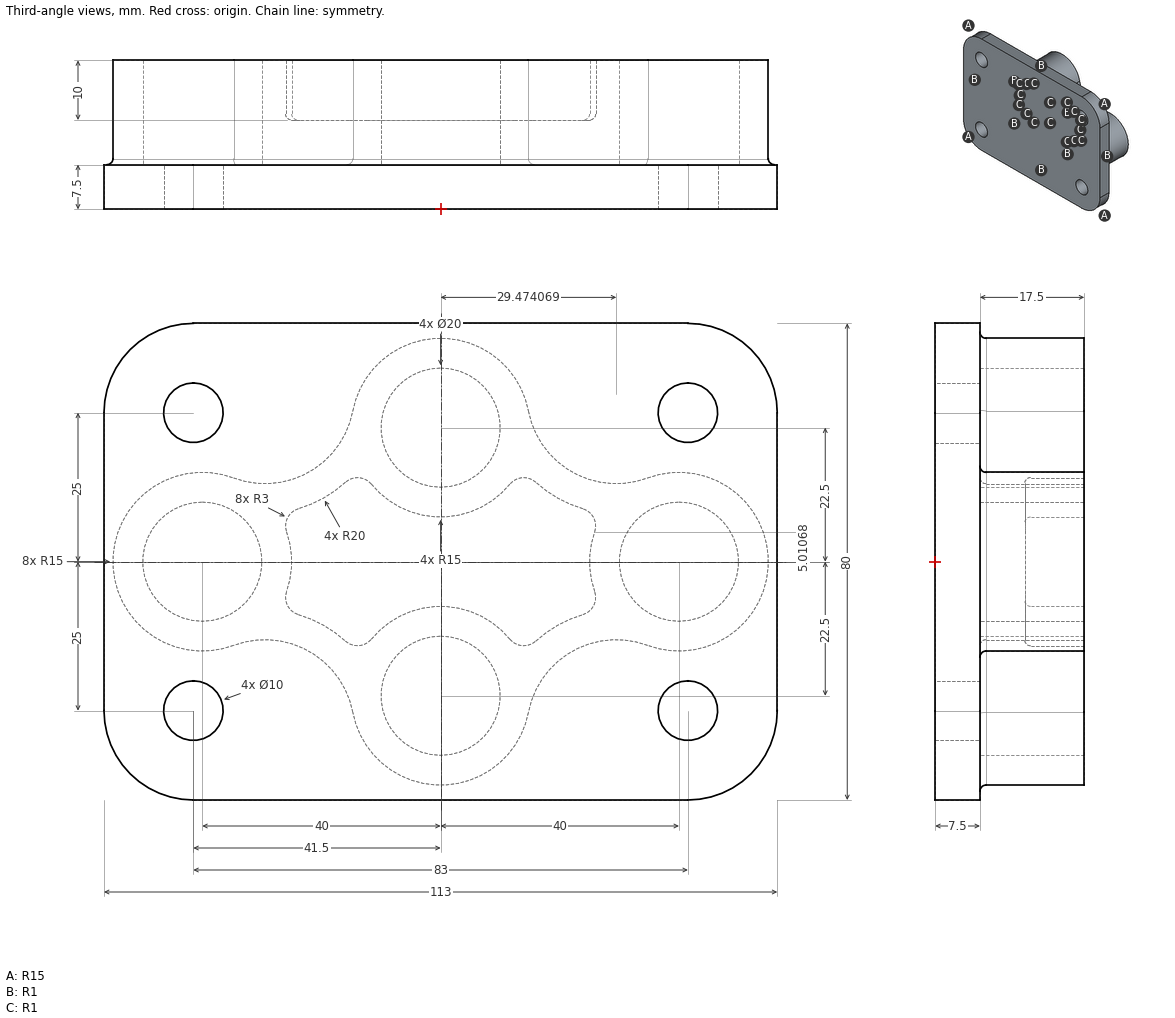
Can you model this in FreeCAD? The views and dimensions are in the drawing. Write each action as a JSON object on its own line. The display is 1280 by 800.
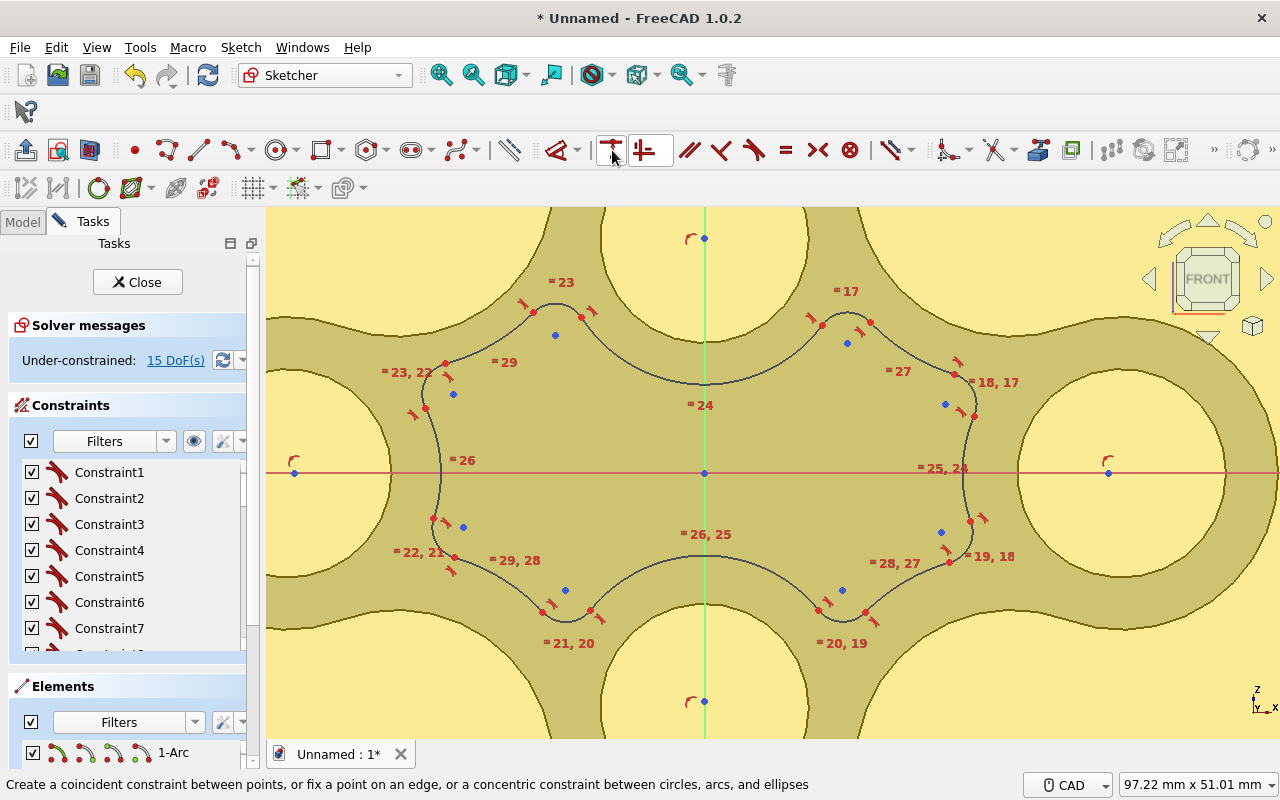
{"action": "scroll", "coordinate": [618, 711], "scroll_direction": "down", "scroll_amount": 1}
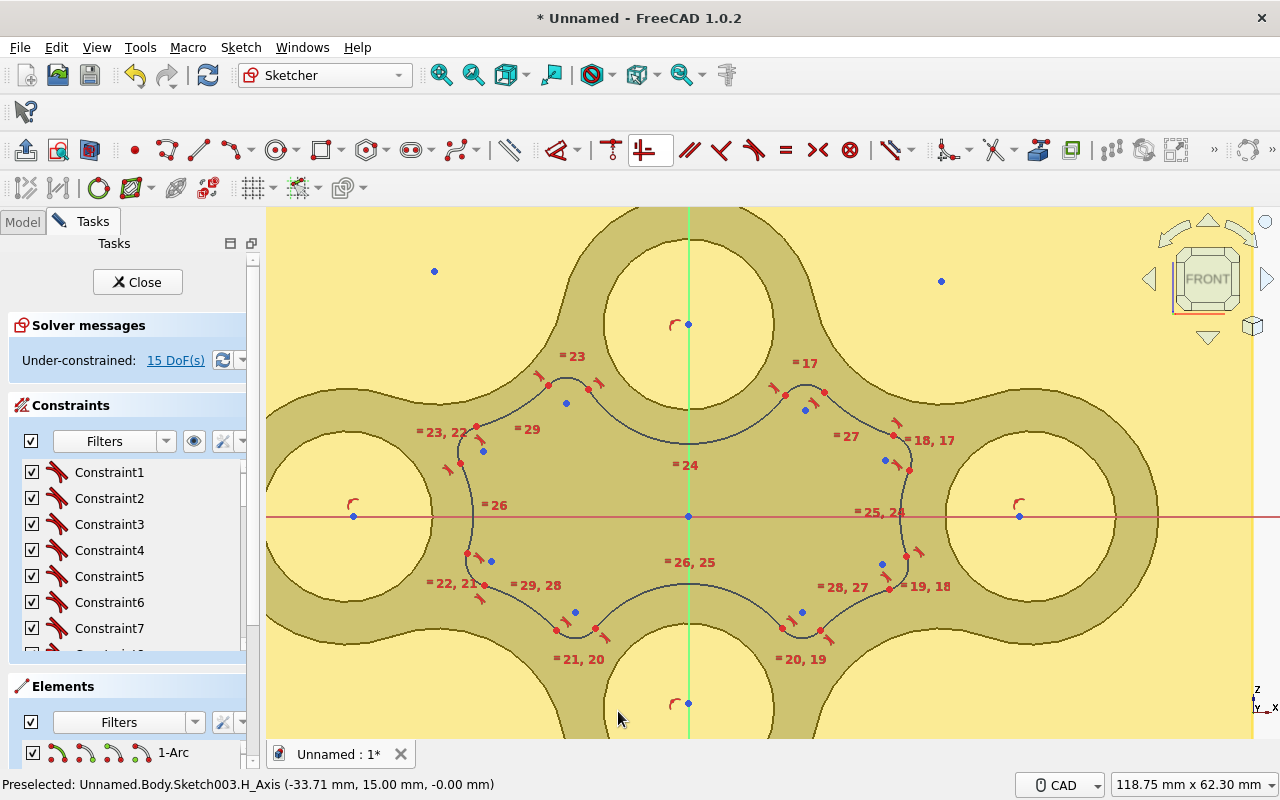
{"action": "left_click", "coordinate": [941, 282]}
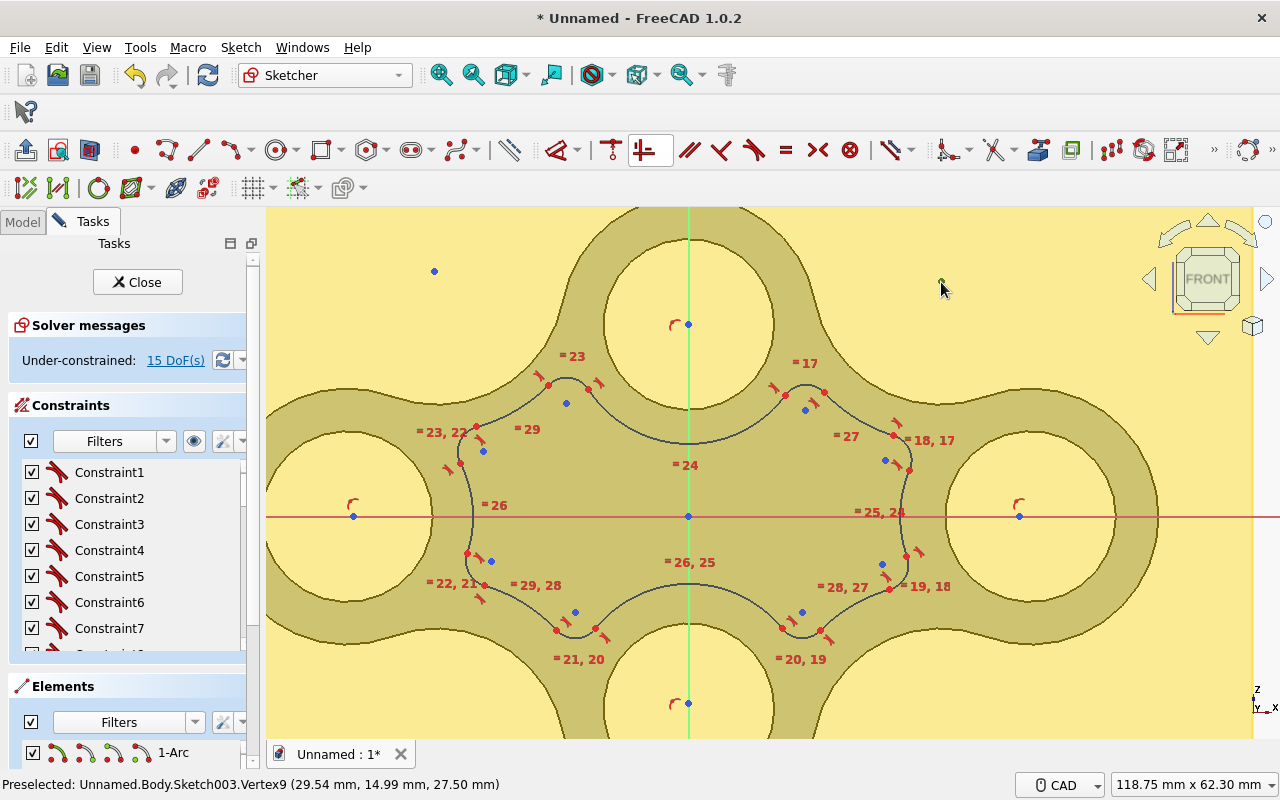
{"action": "scroll", "coordinate": [719, 235], "scroll_direction": "down", "scroll_amount": 1}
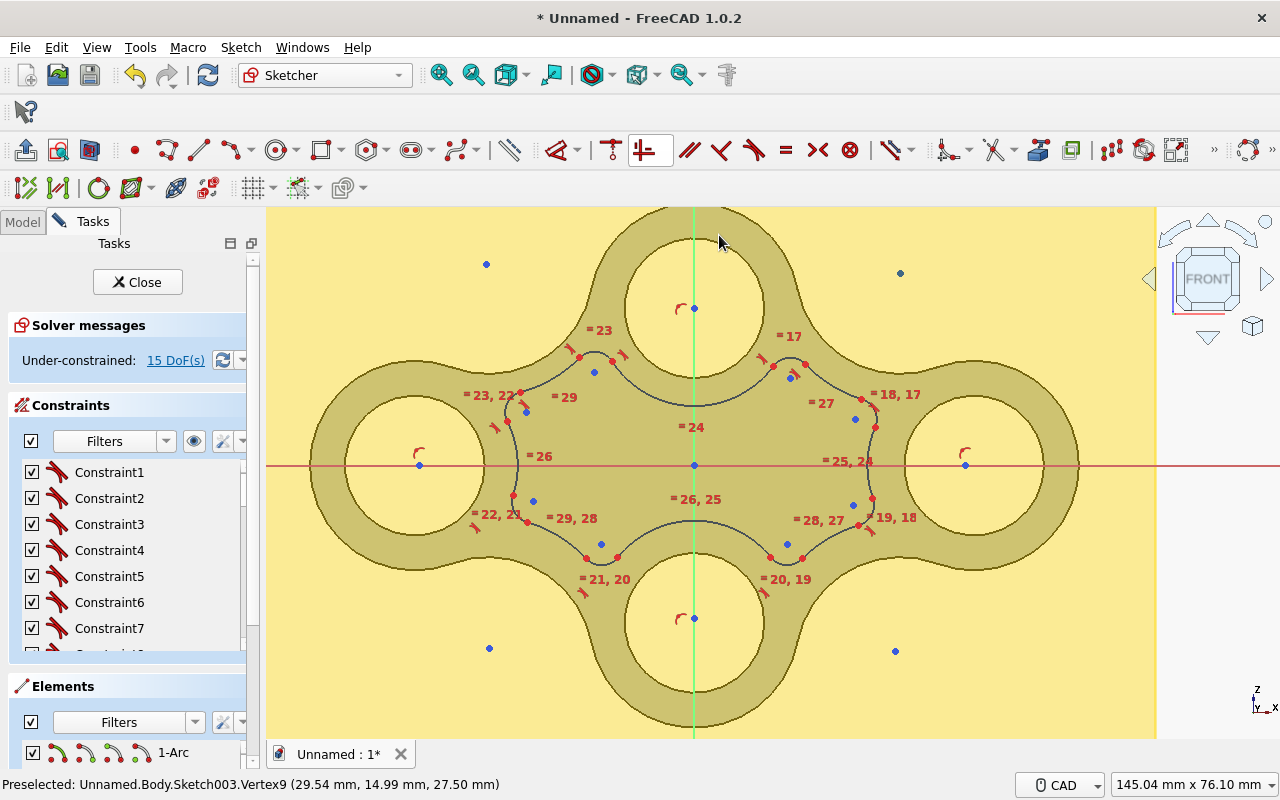
{"action": "left_click", "coordinate": [896, 652]}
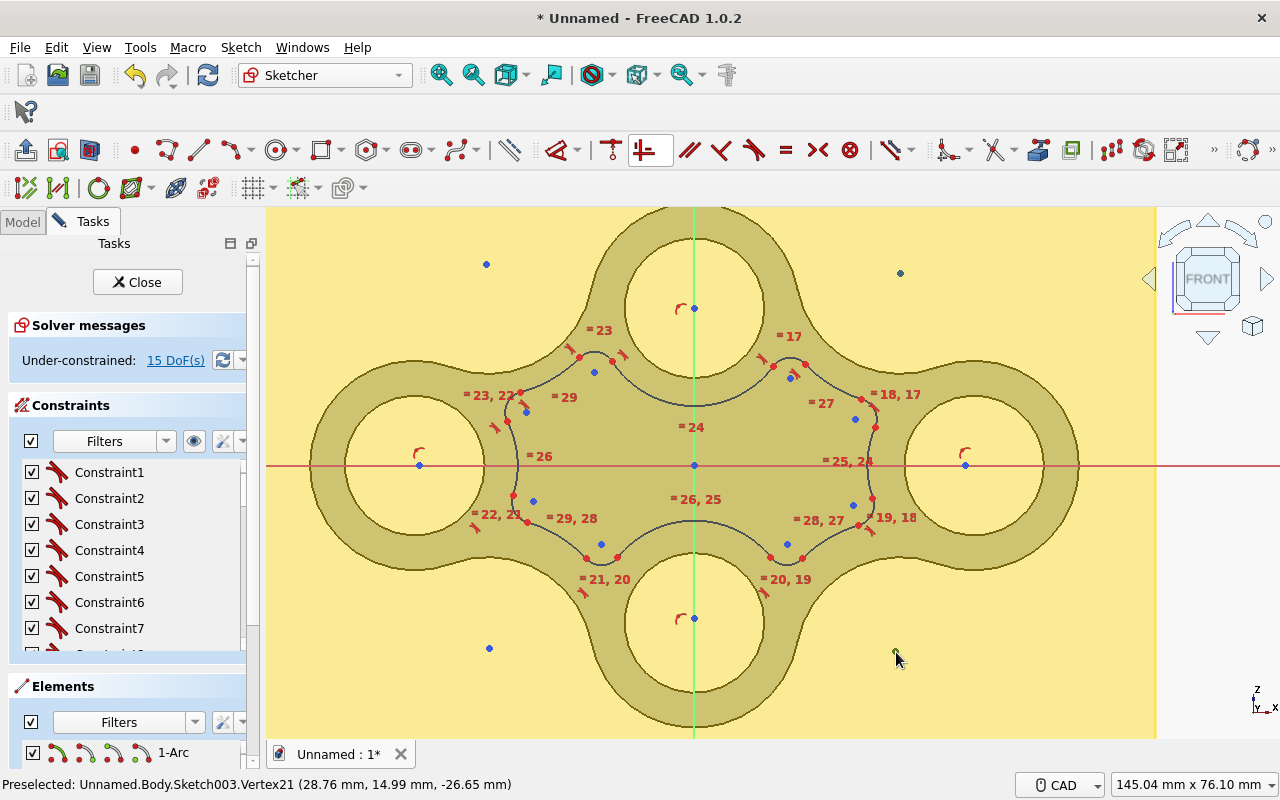
{"action": "left_click", "coordinate": [353, 466]}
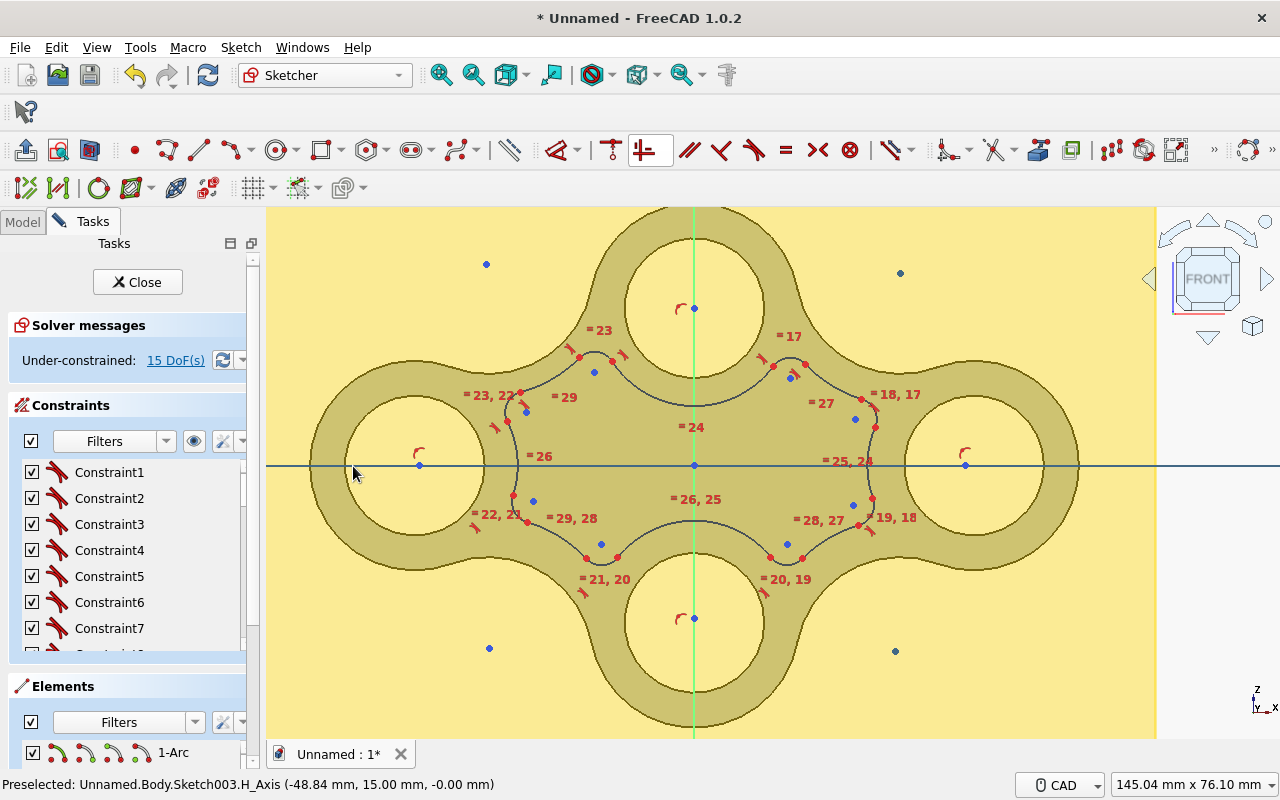
{"action": "key", "text": "s"}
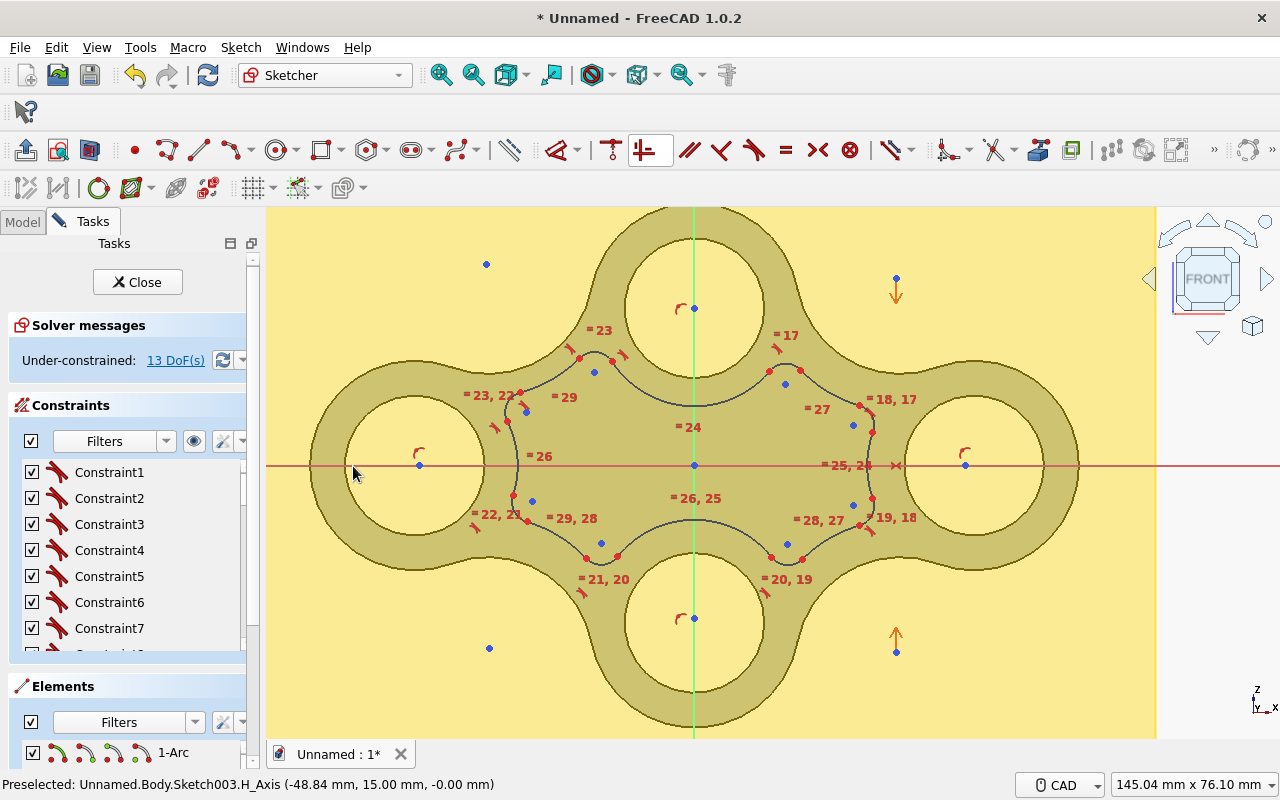
{"action": "left_click", "coordinate": [896, 652]}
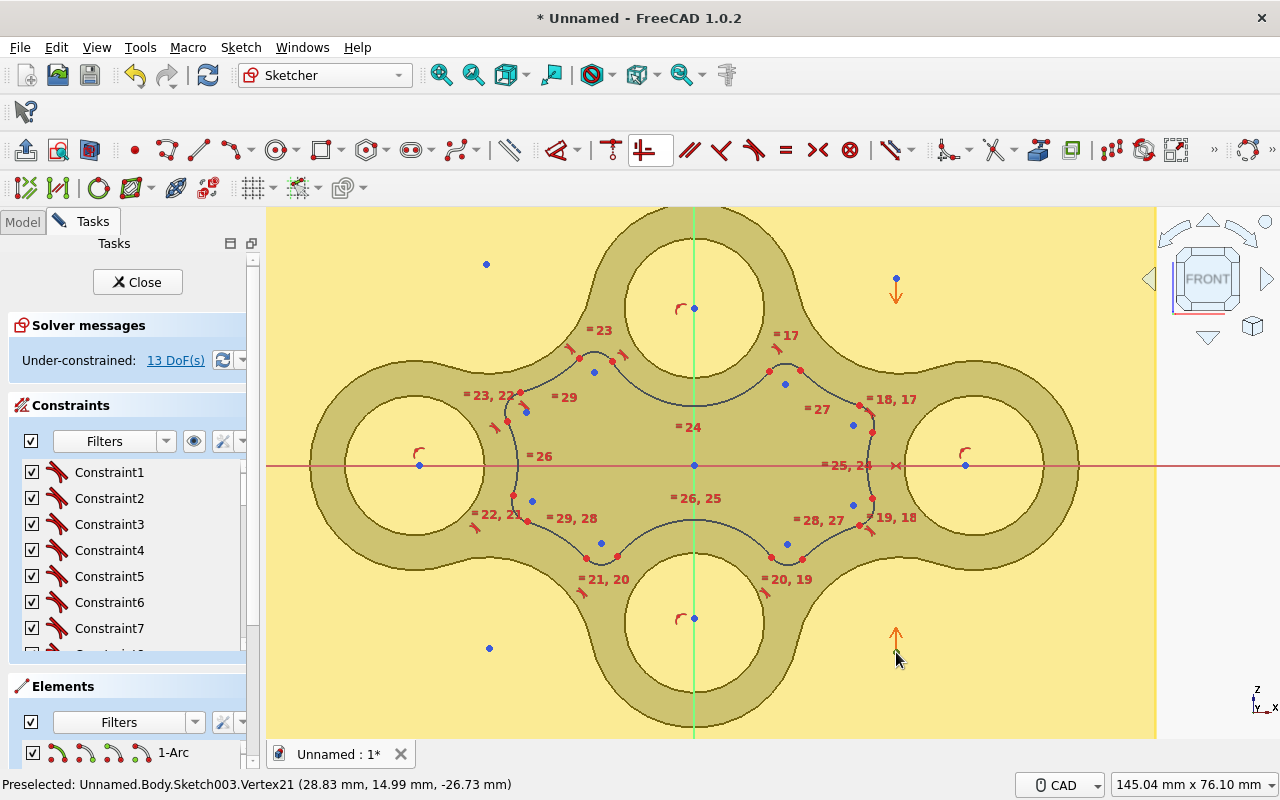
{"action": "left_click", "coordinate": [490, 649]}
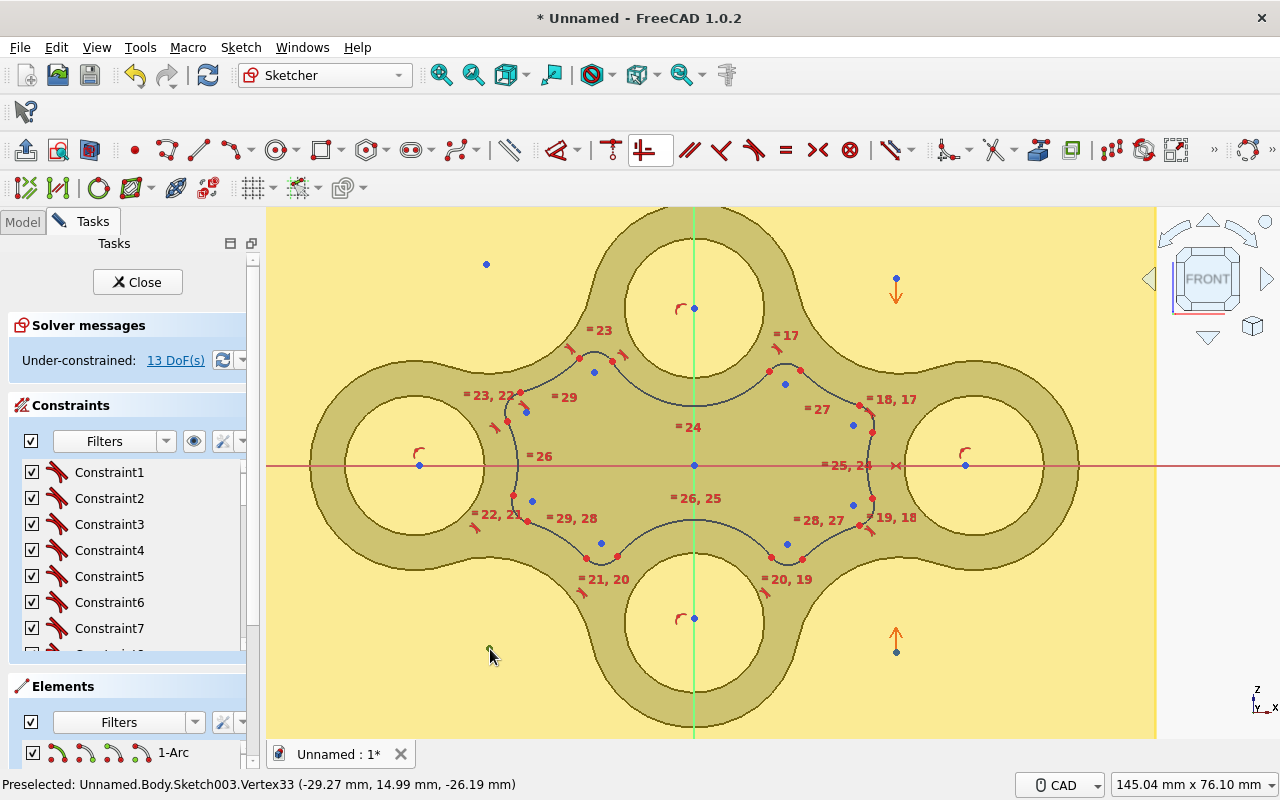
{"action": "left_click", "coordinate": [694, 677]}